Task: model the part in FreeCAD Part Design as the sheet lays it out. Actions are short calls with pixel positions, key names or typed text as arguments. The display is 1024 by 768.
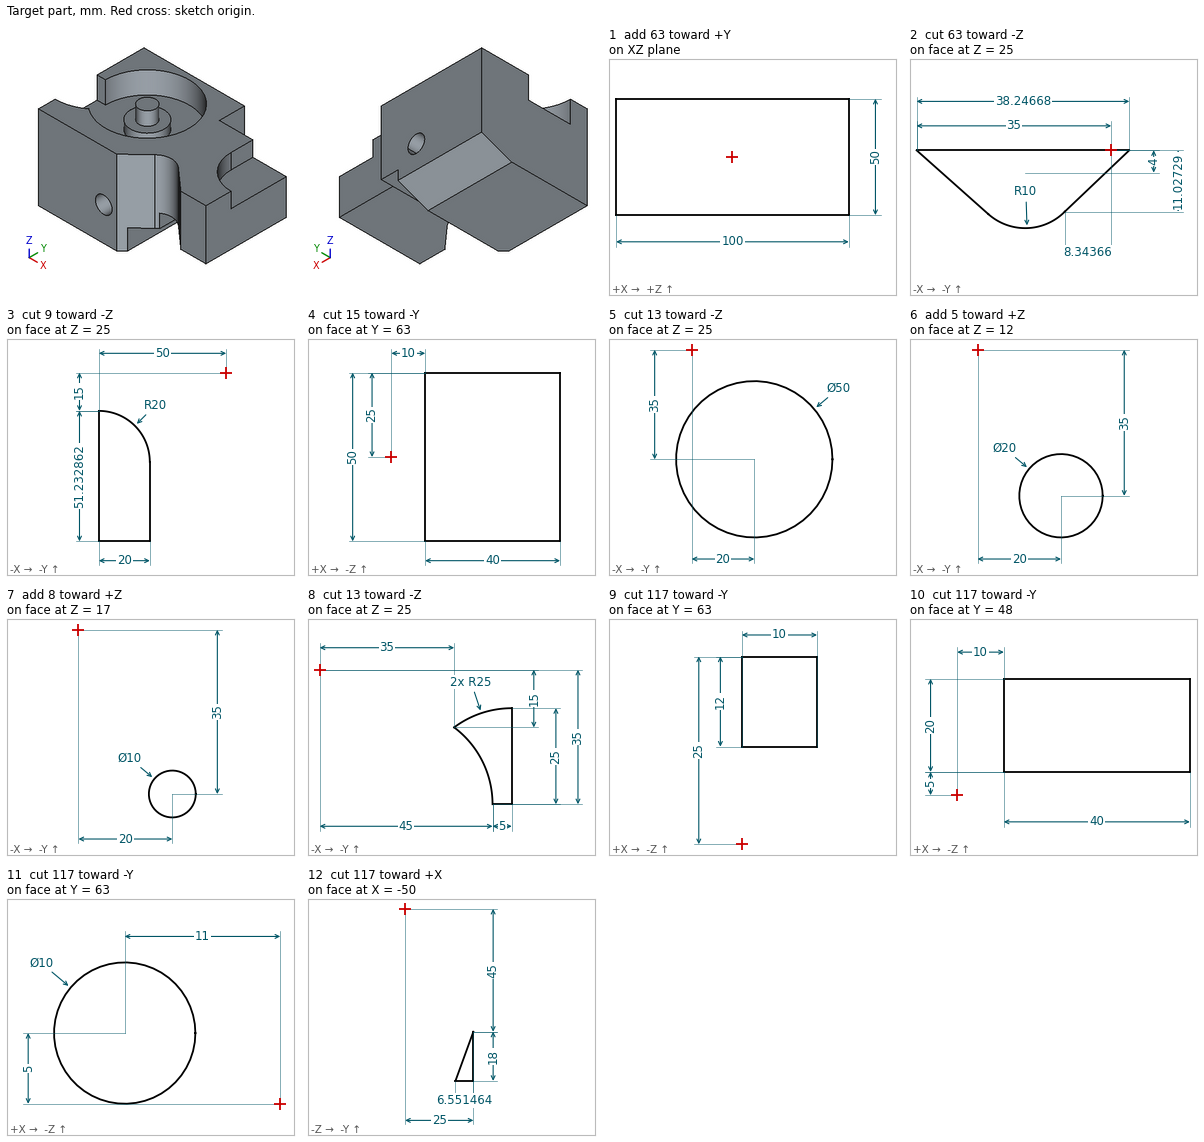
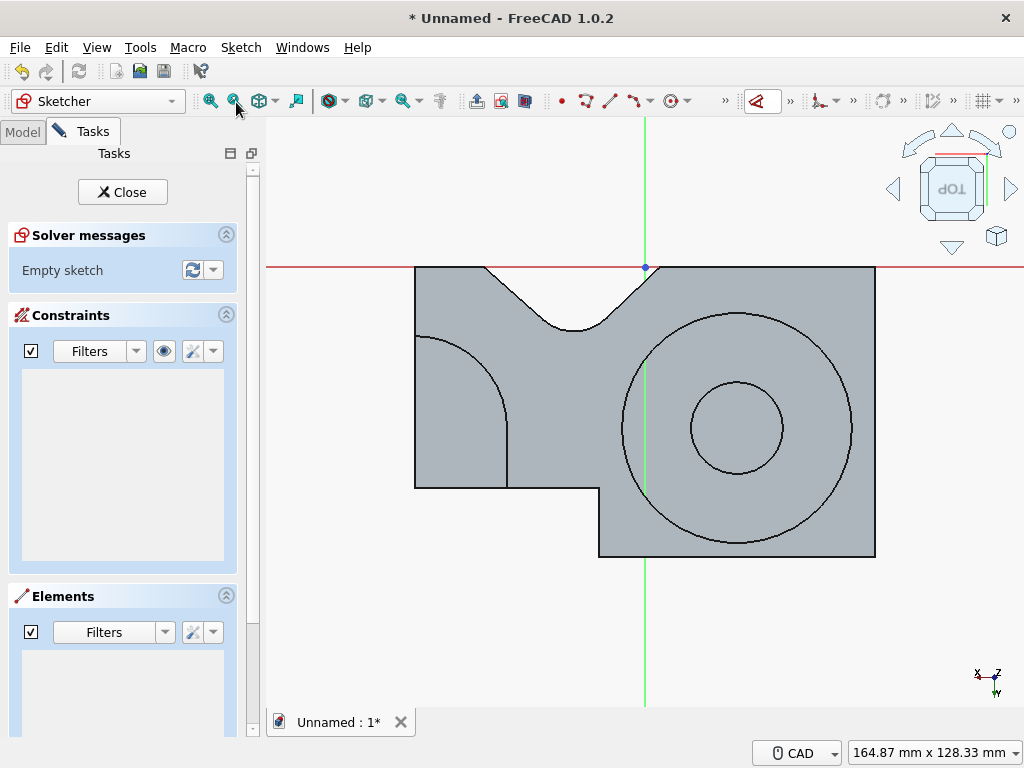
click(526, 102)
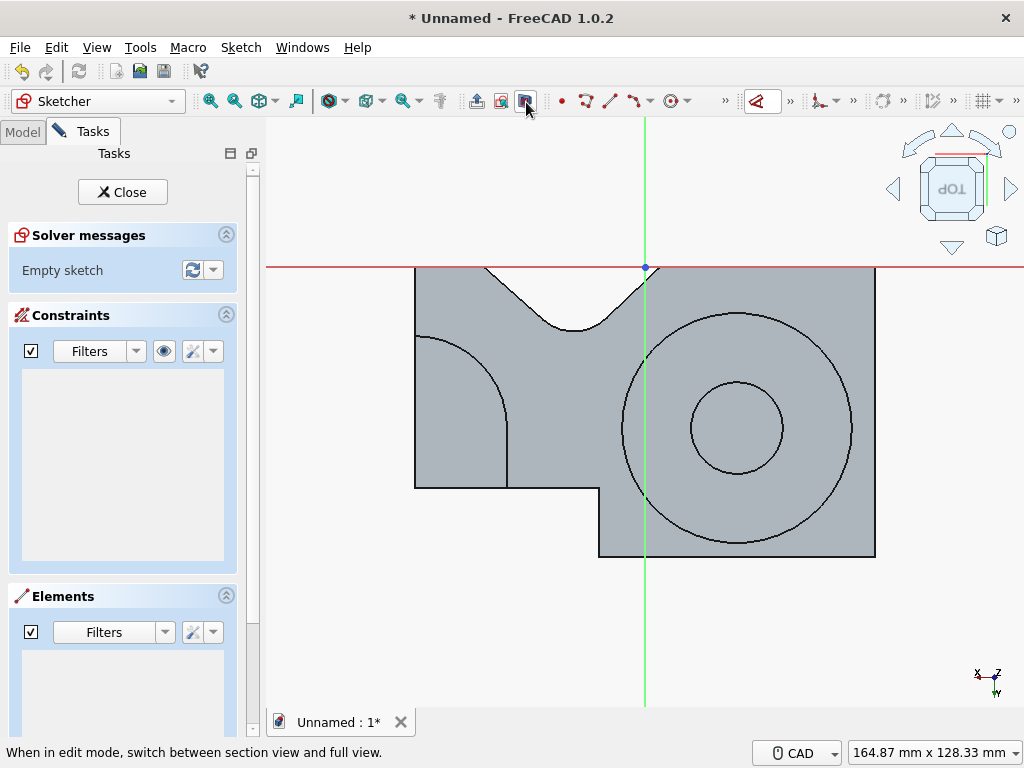
scroll(757, 430, up, 11)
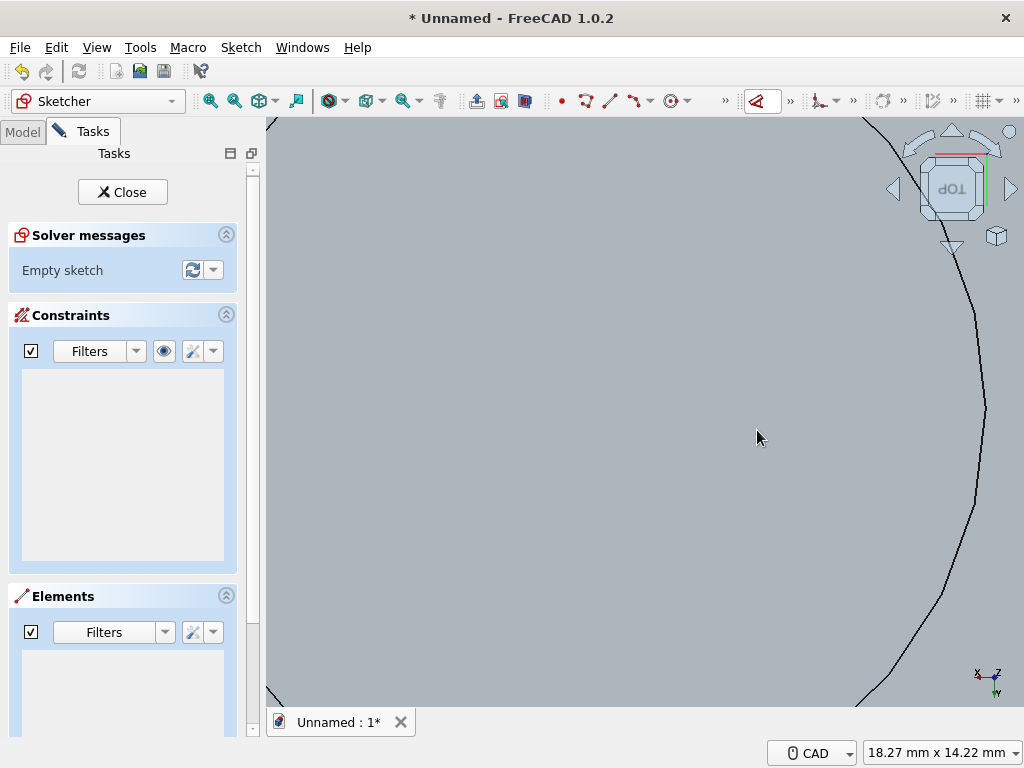
click(672, 102)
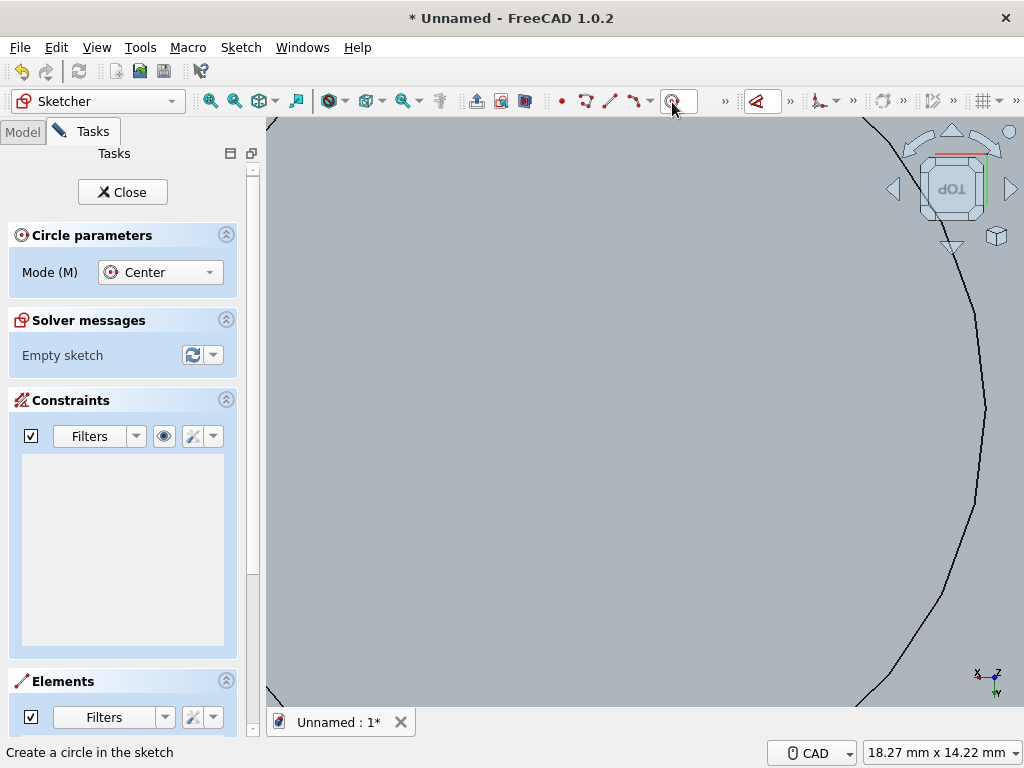
click(571, 409)
click(718, 262)
key(Escape)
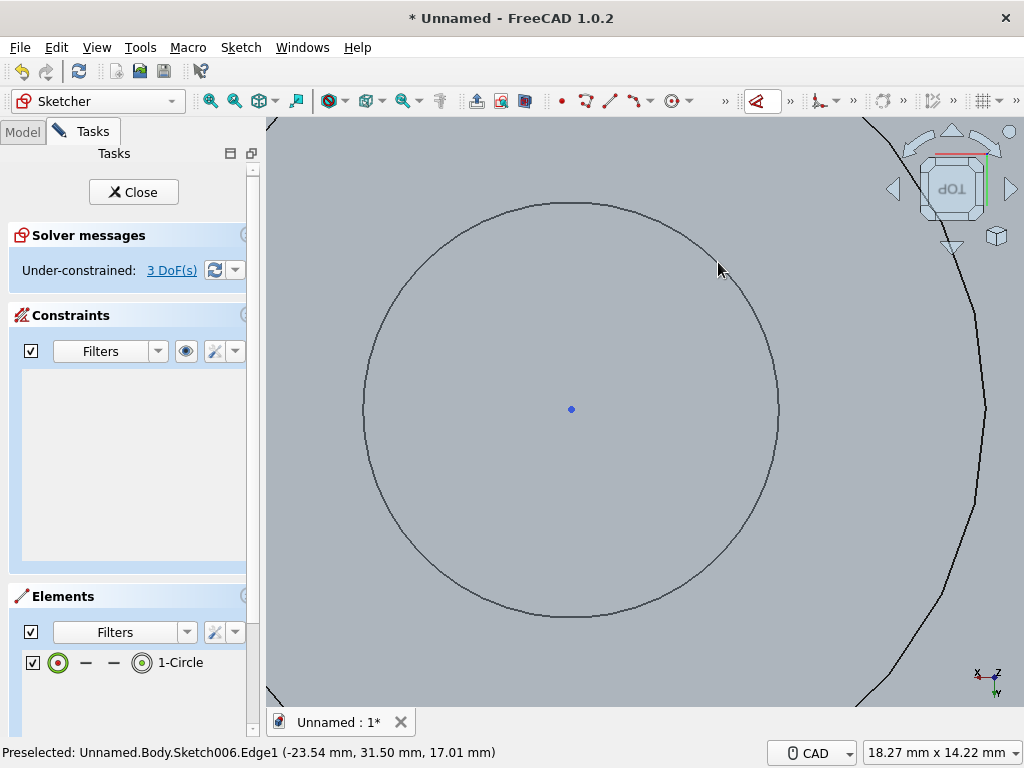
click(718, 263)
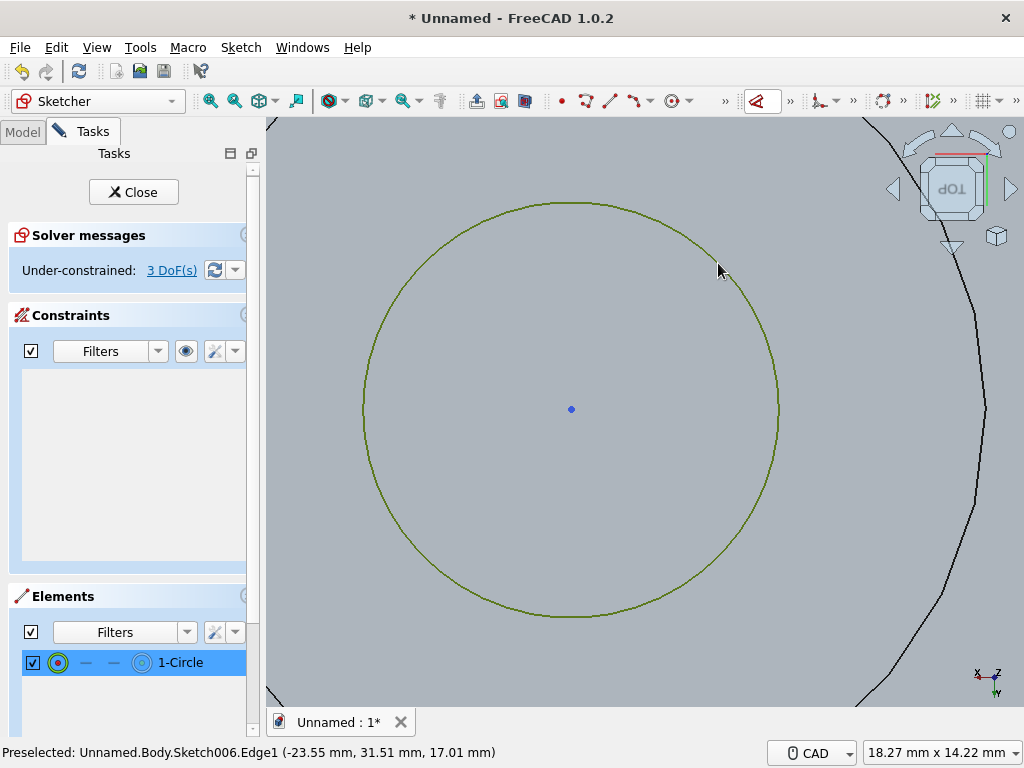
click(776, 102)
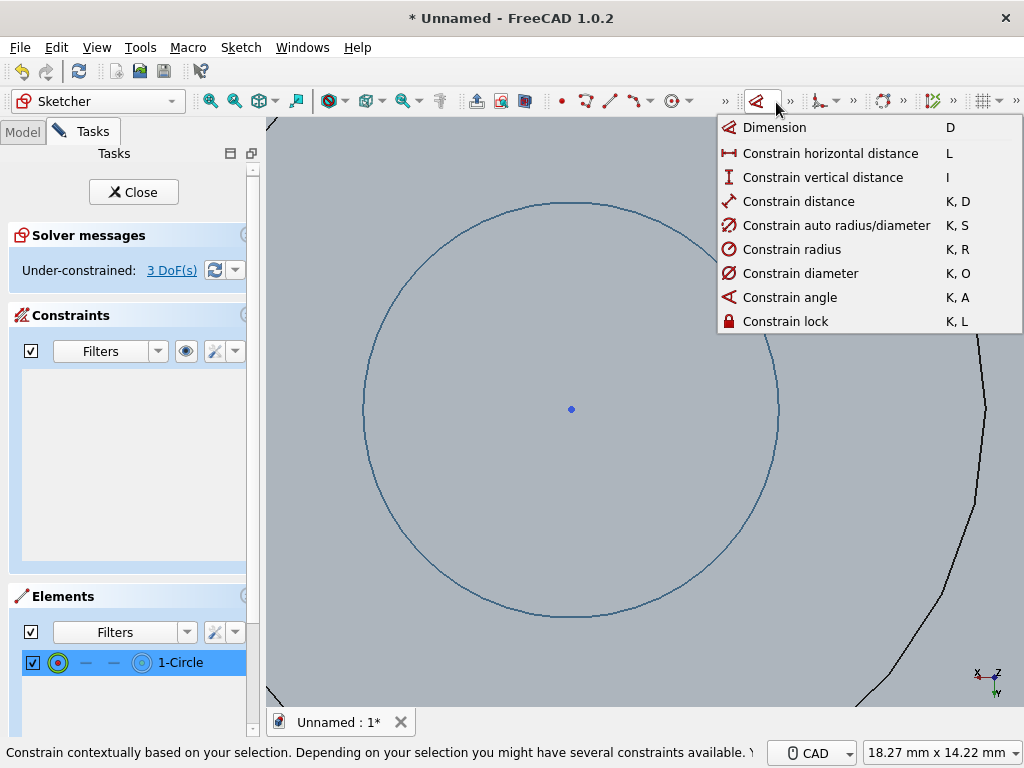
click(870, 273)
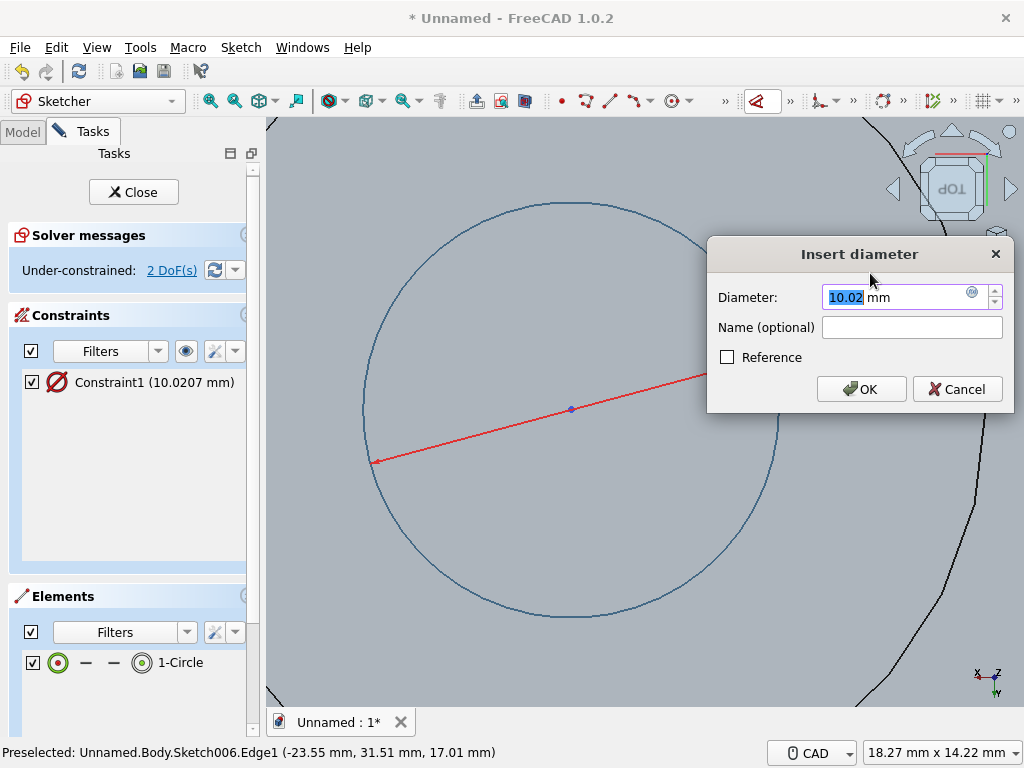
text(10)
key(Return)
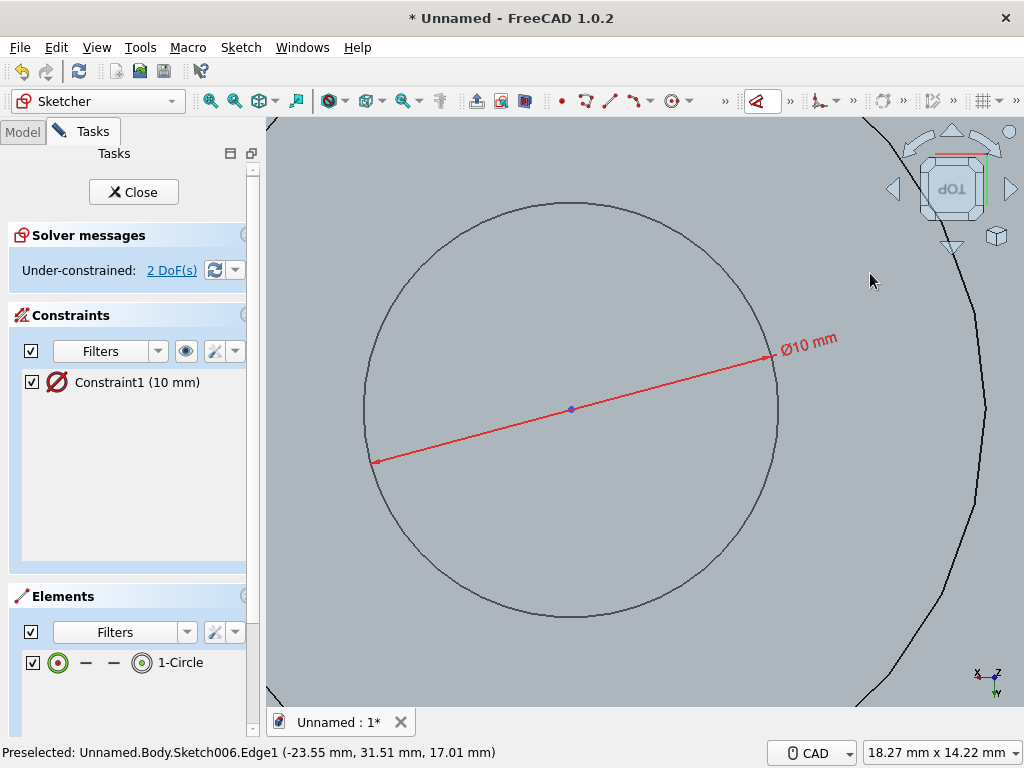
click(571, 410)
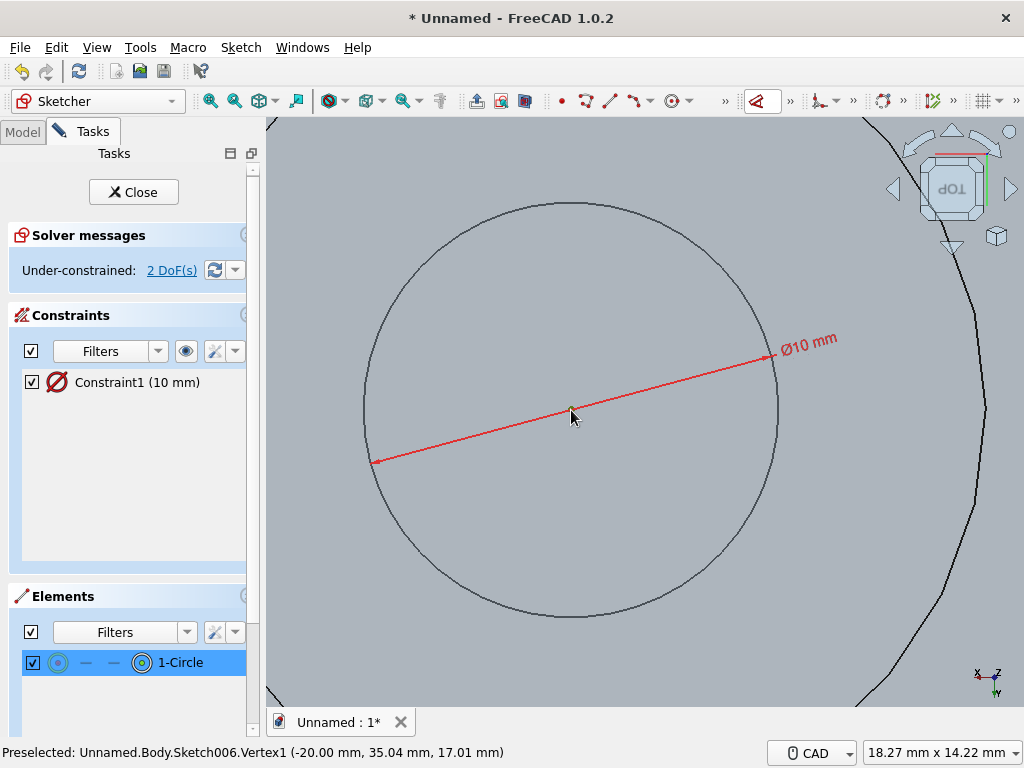
click(776, 102)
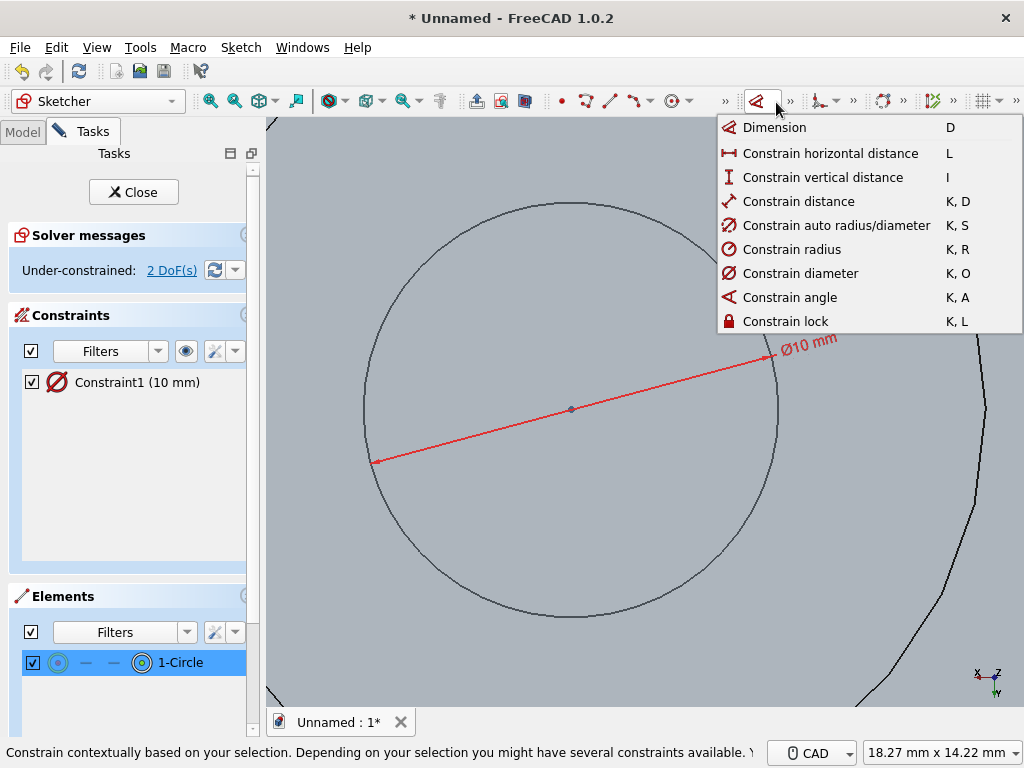
click(870, 153)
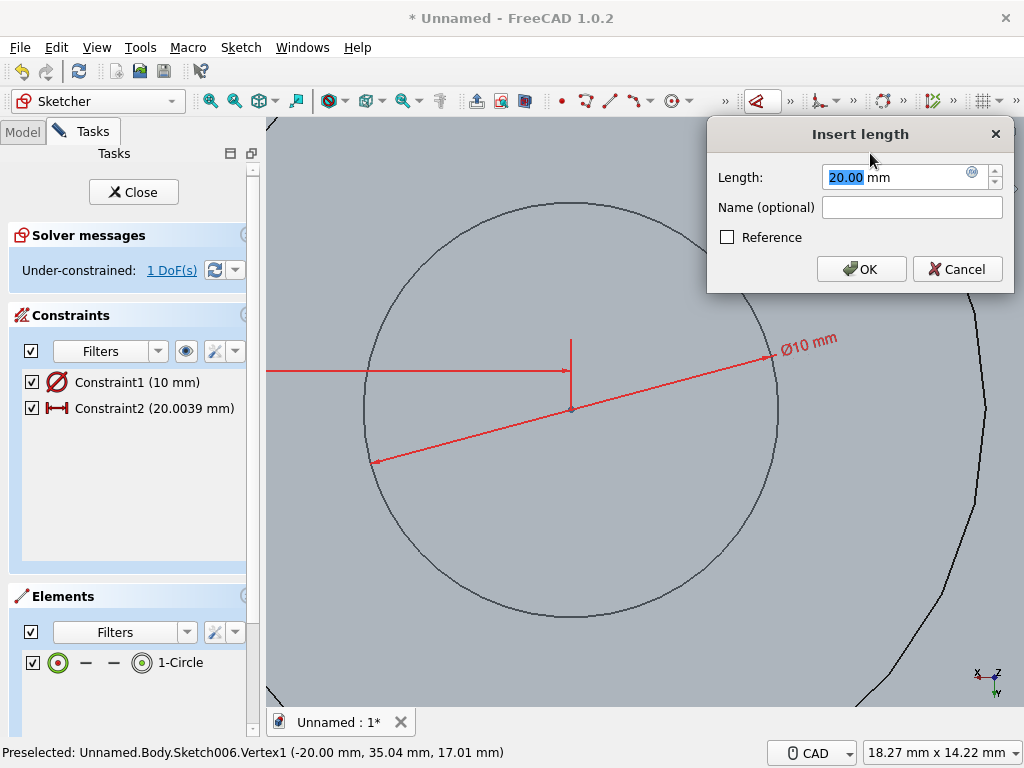
text(20)
key(Return)